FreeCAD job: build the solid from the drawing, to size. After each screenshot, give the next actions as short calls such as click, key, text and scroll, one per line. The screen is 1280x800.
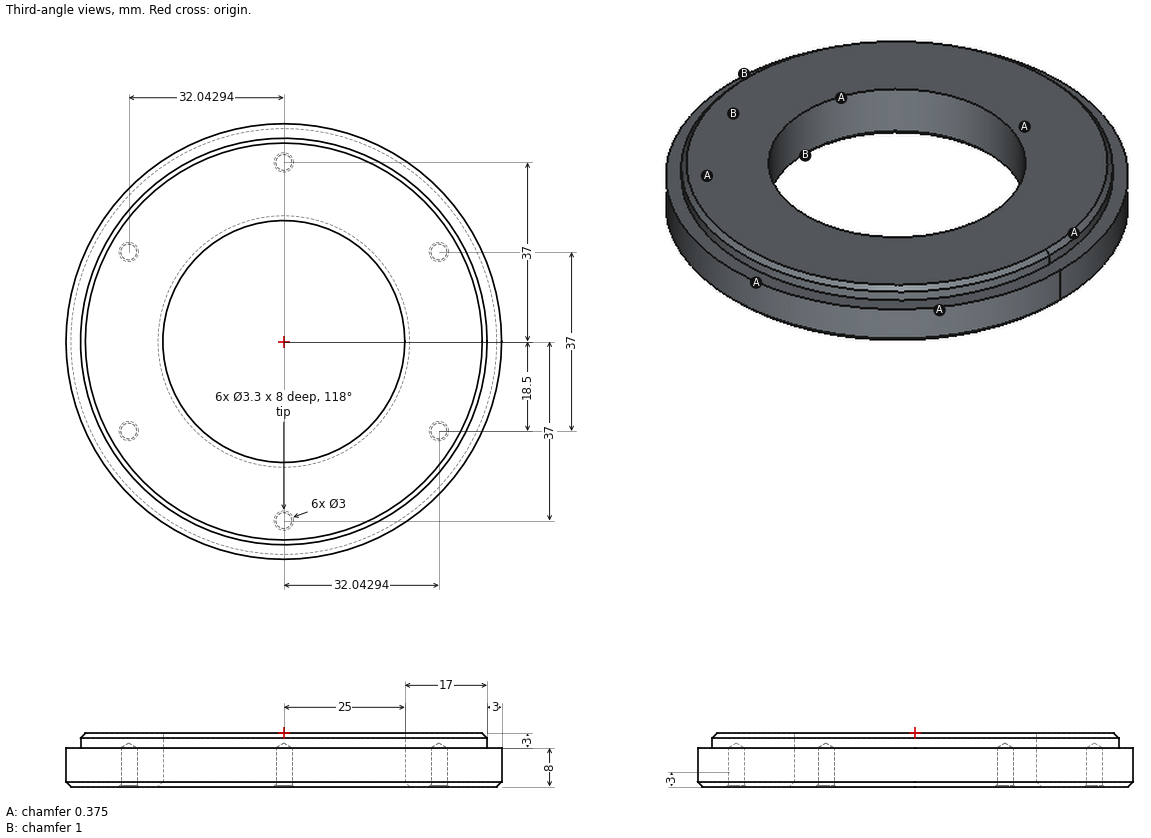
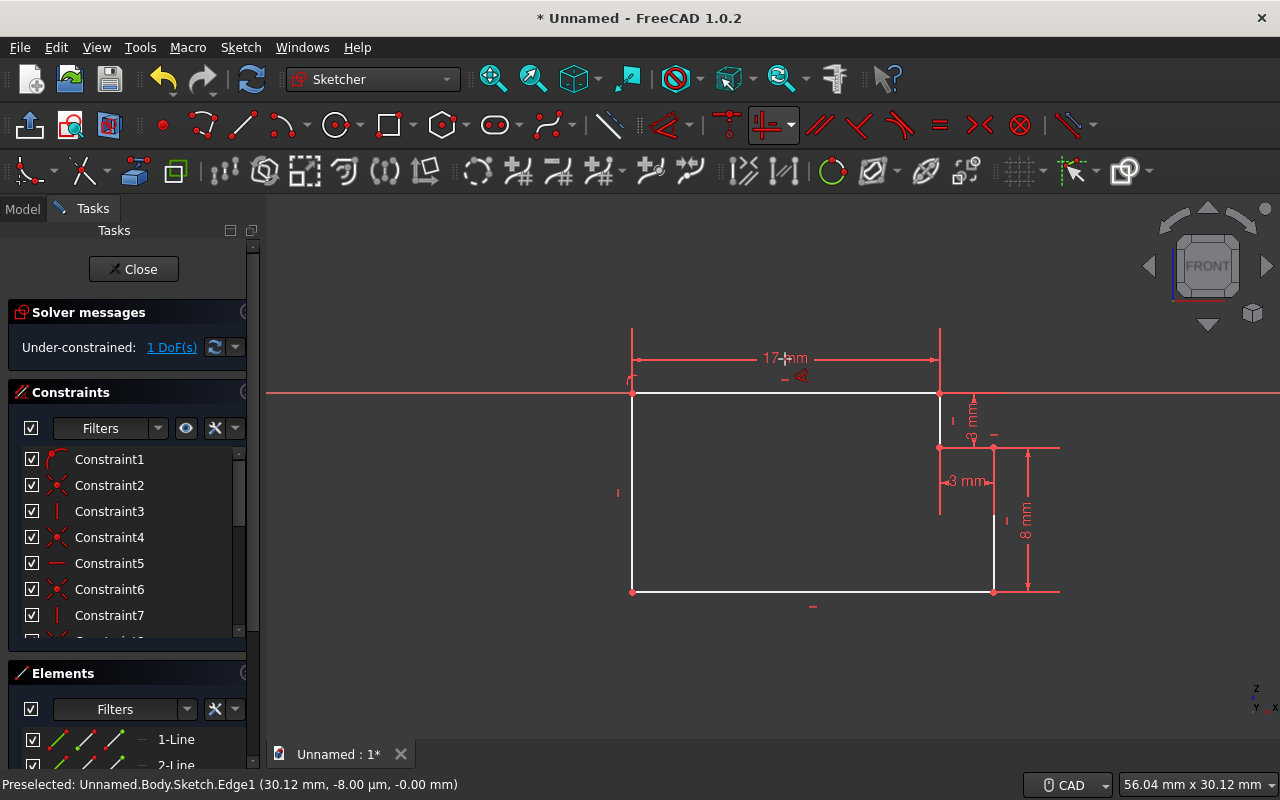
click(632, 393)
click(463, 359)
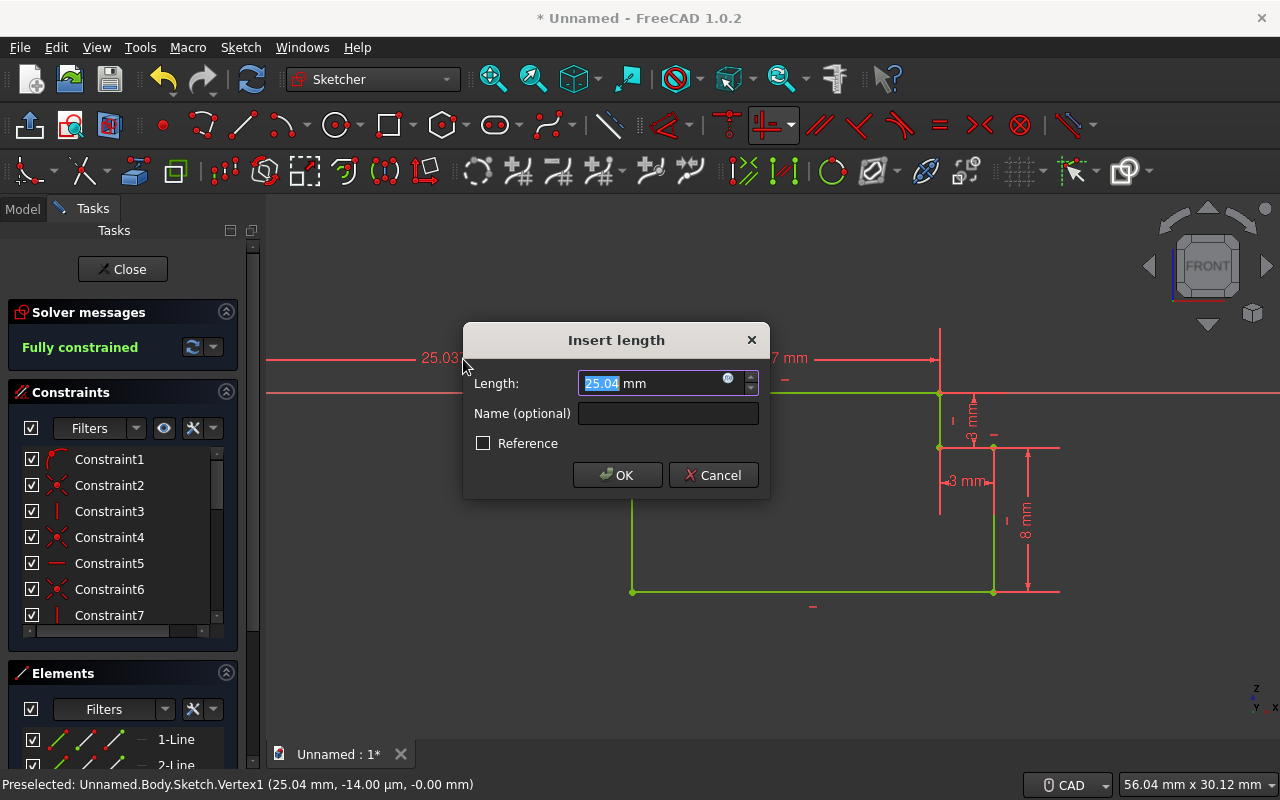
text(25)
key(Return)
key(Escape)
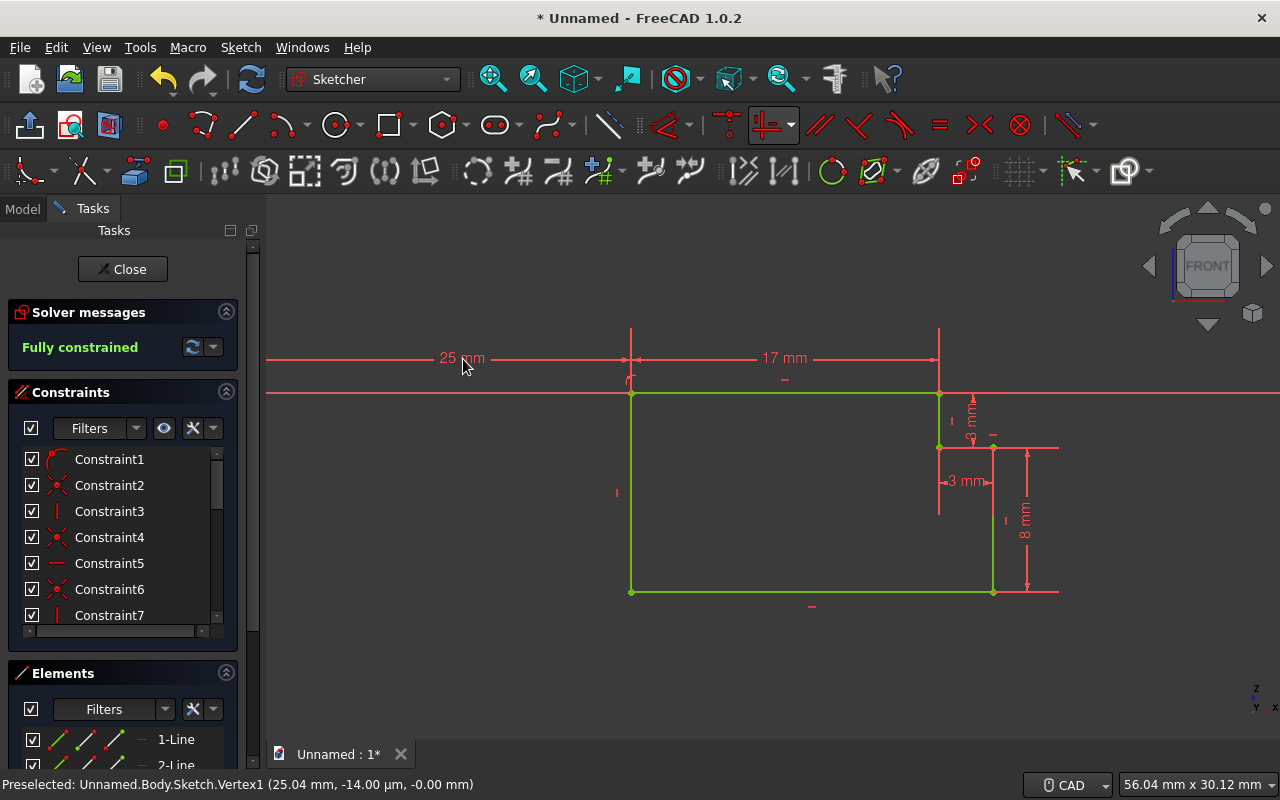
click(123, 269)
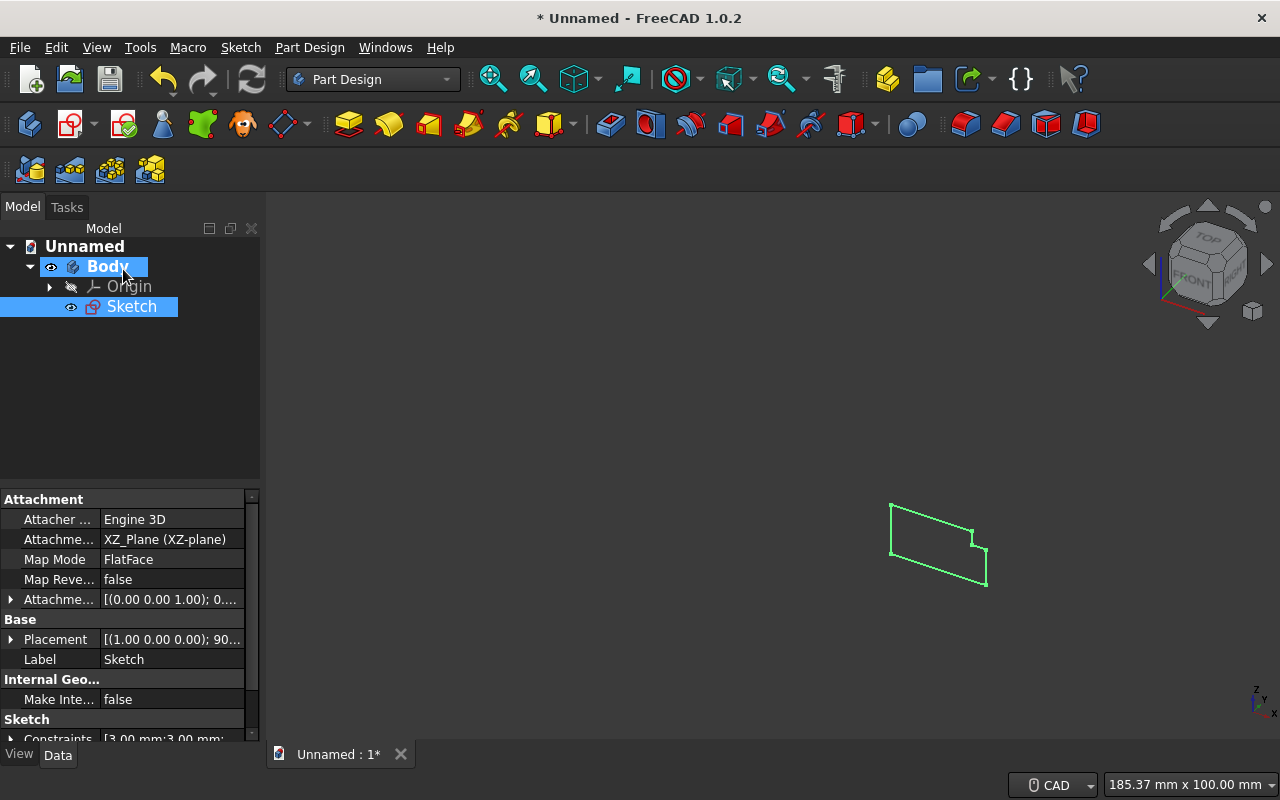
click(390, 124)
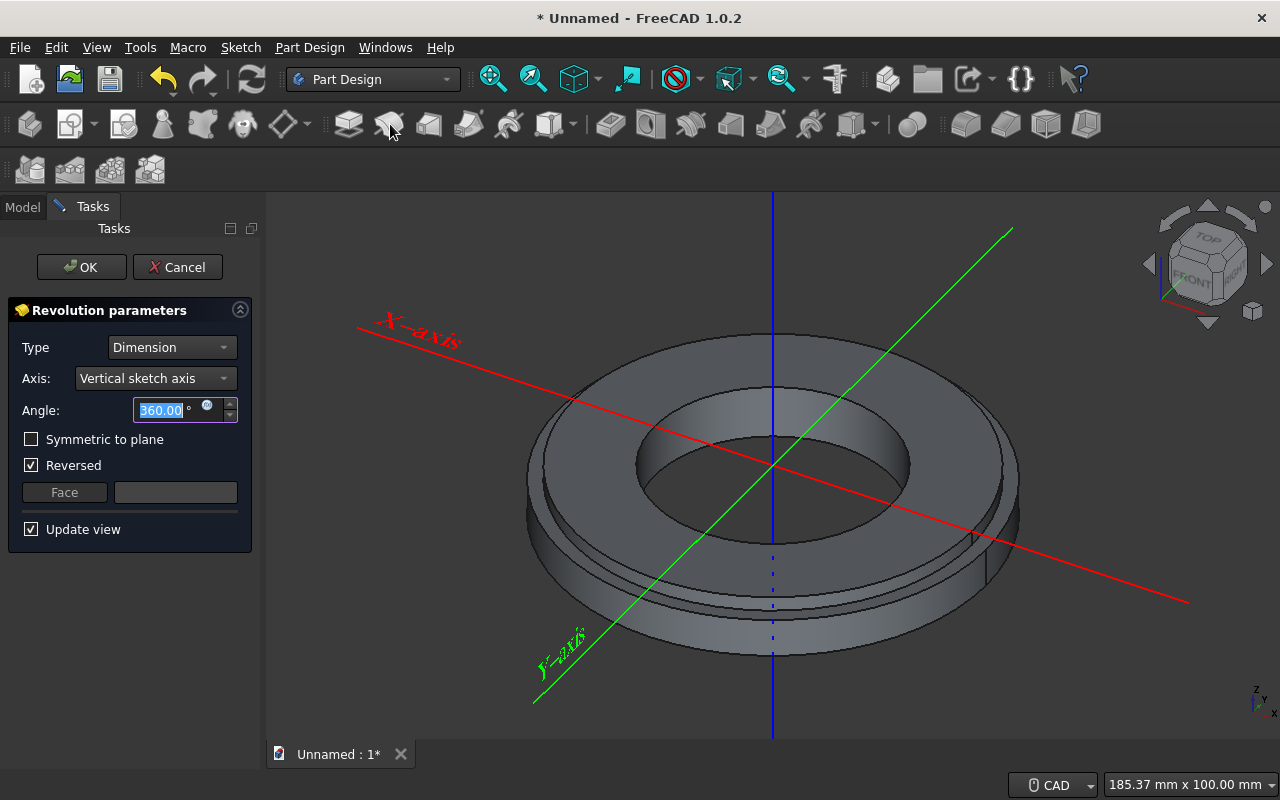
click(82, 267)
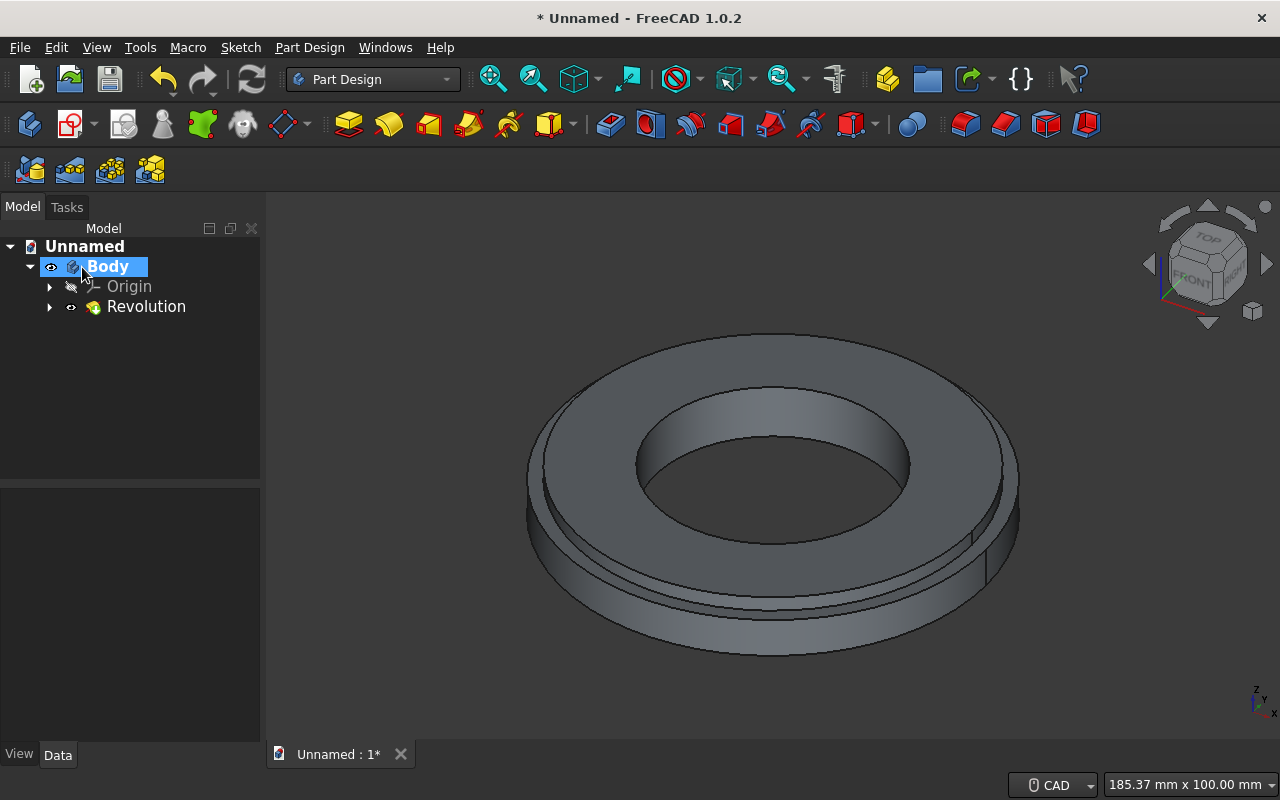
key(5)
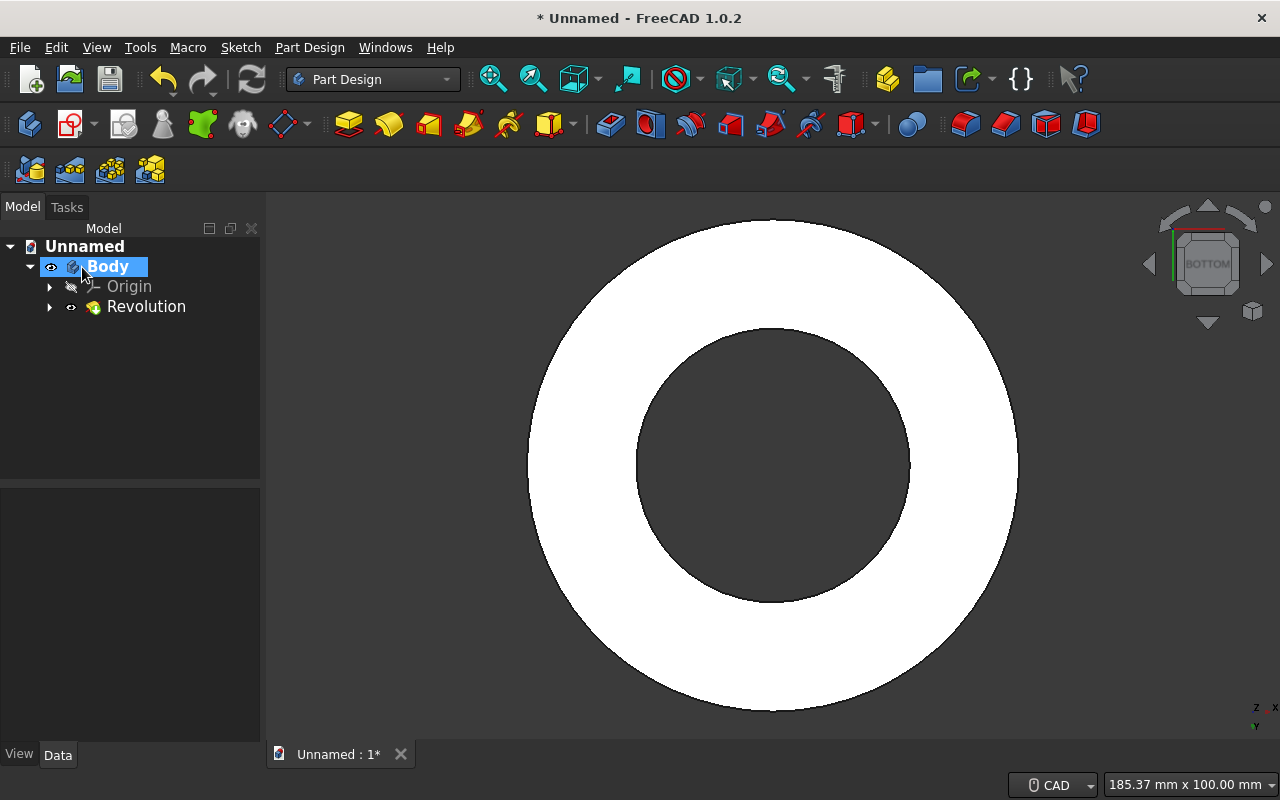
click(914, 324)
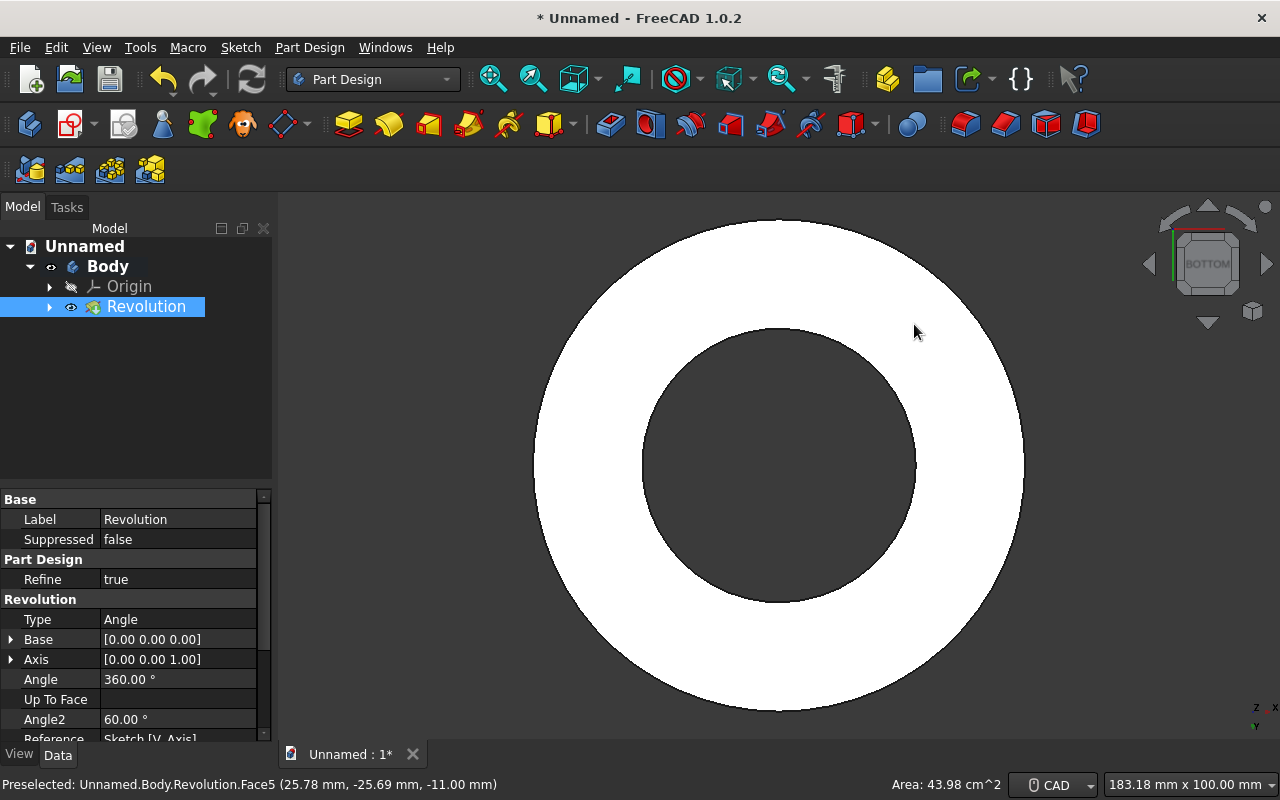
click(70, 124)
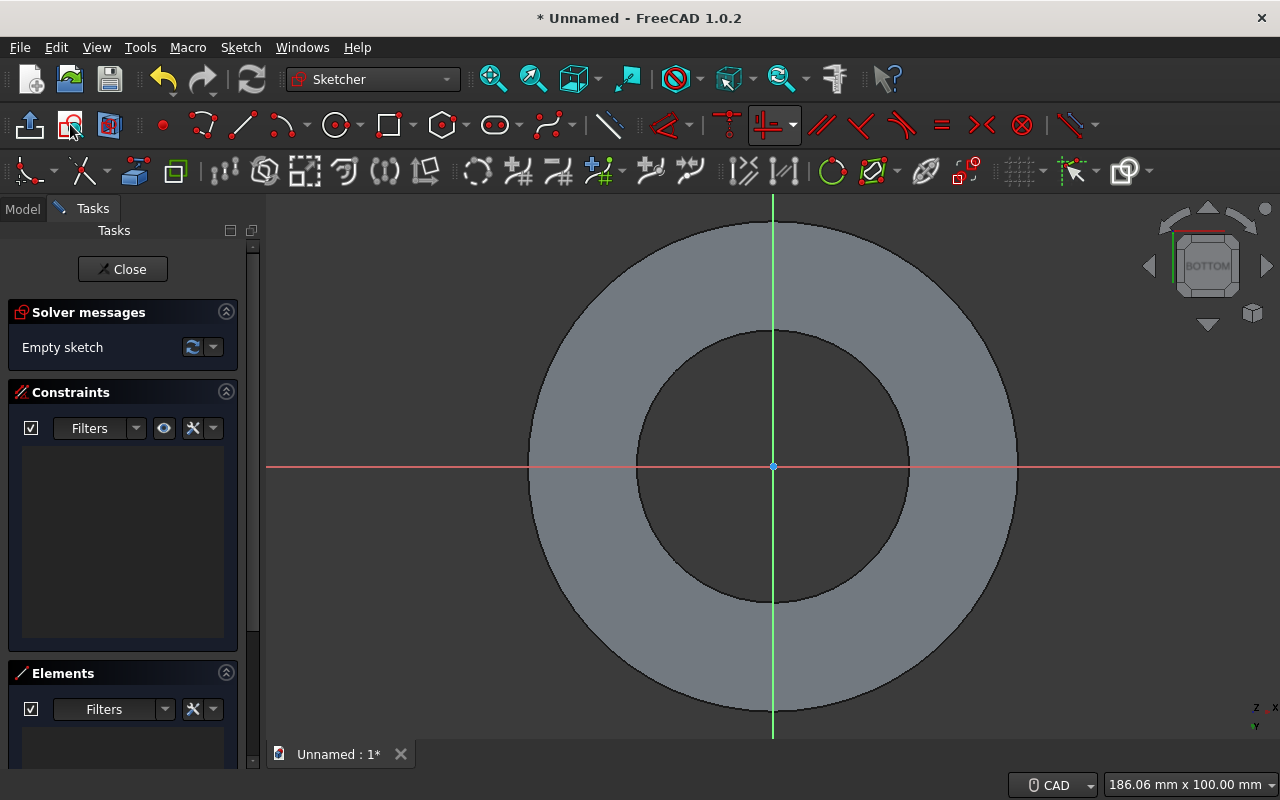
click(336, 126)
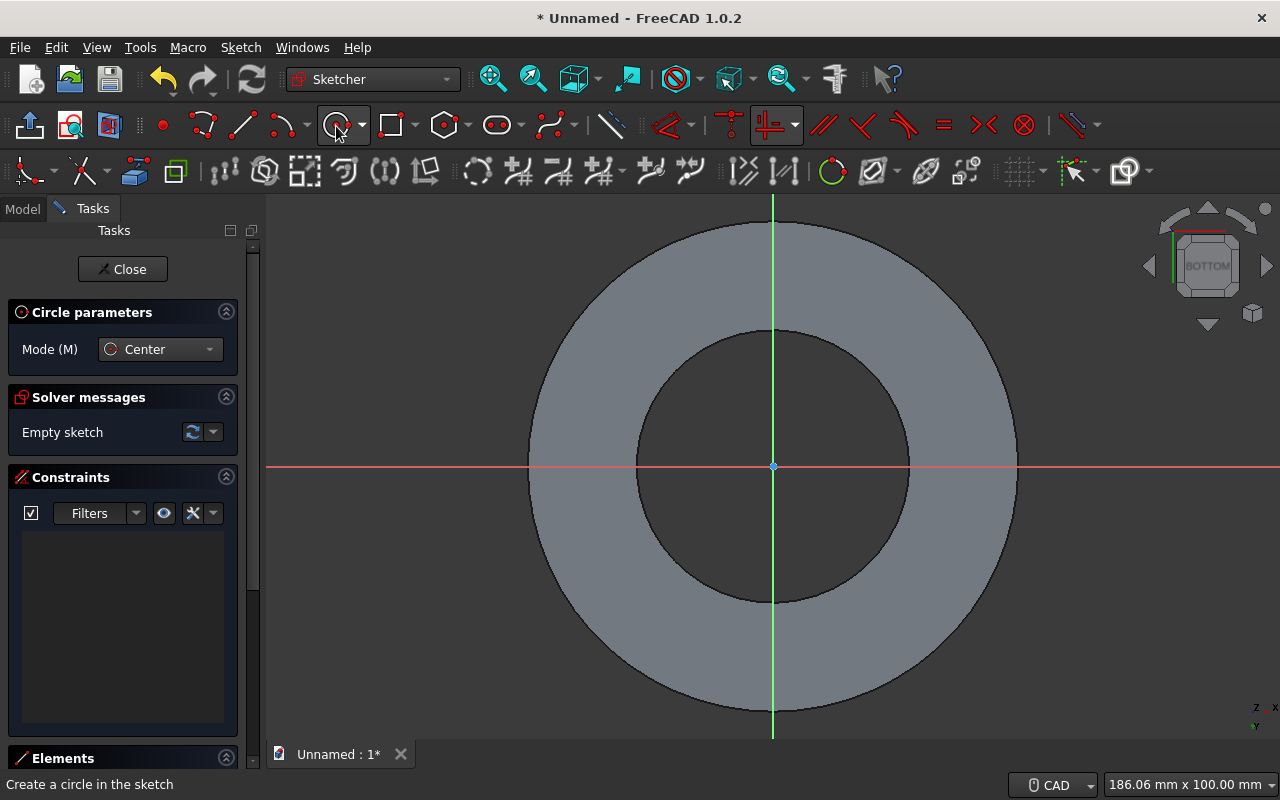
scroll(773, 265, up, 6)